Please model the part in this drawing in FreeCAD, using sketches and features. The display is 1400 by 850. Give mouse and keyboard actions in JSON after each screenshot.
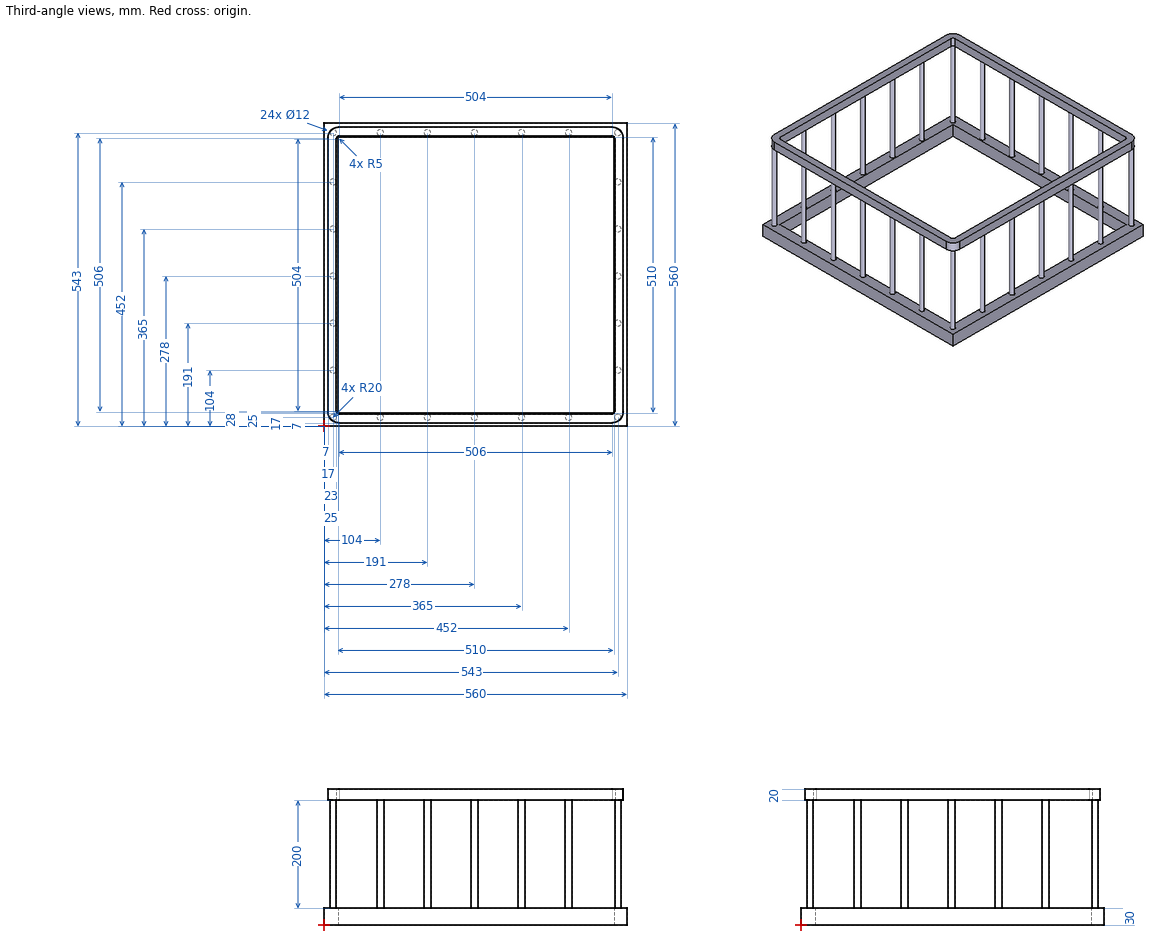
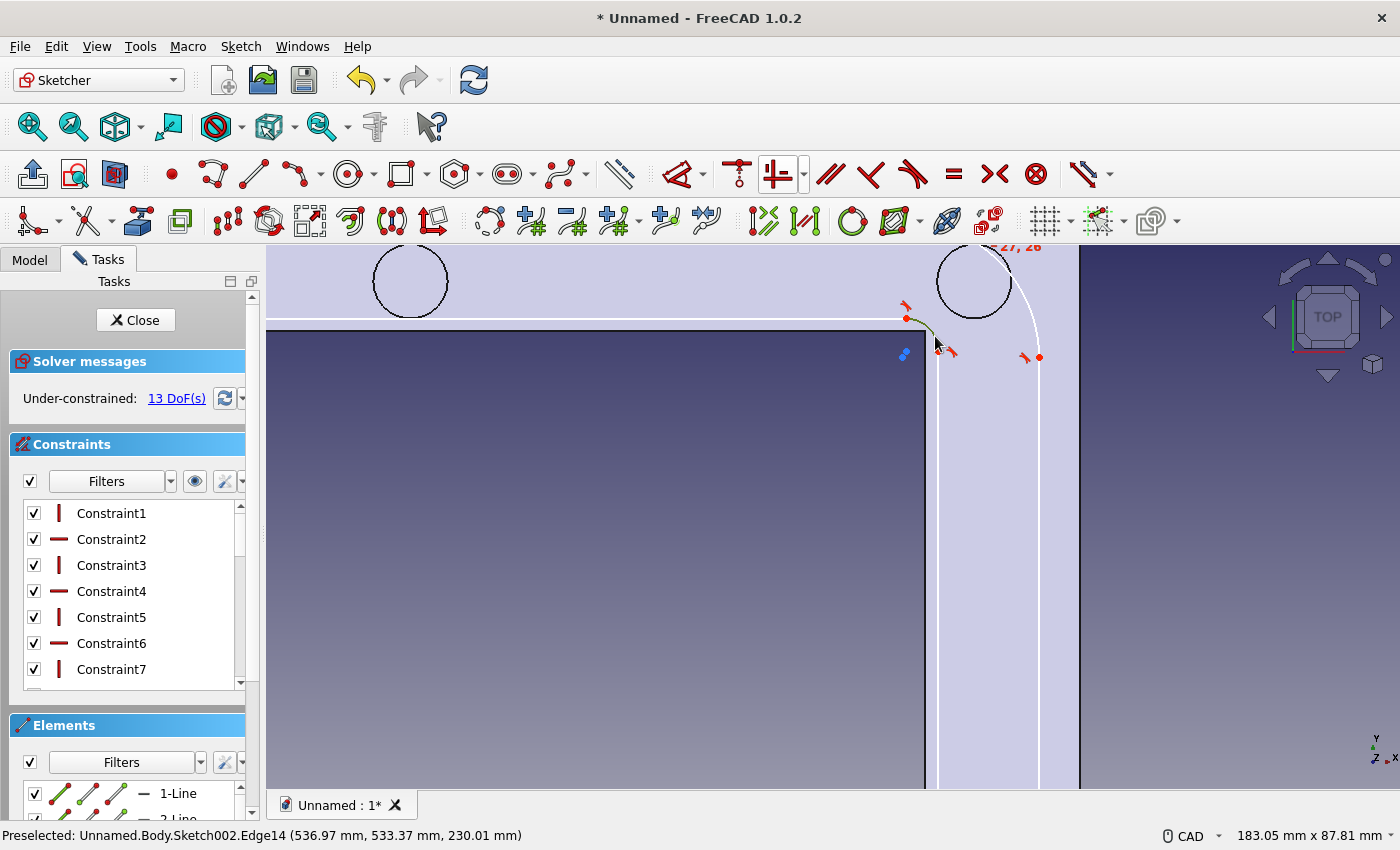
{"action": "scroll", "coordinate": [944, 341], "scroll_direction": "down", "scroll_amount": 11}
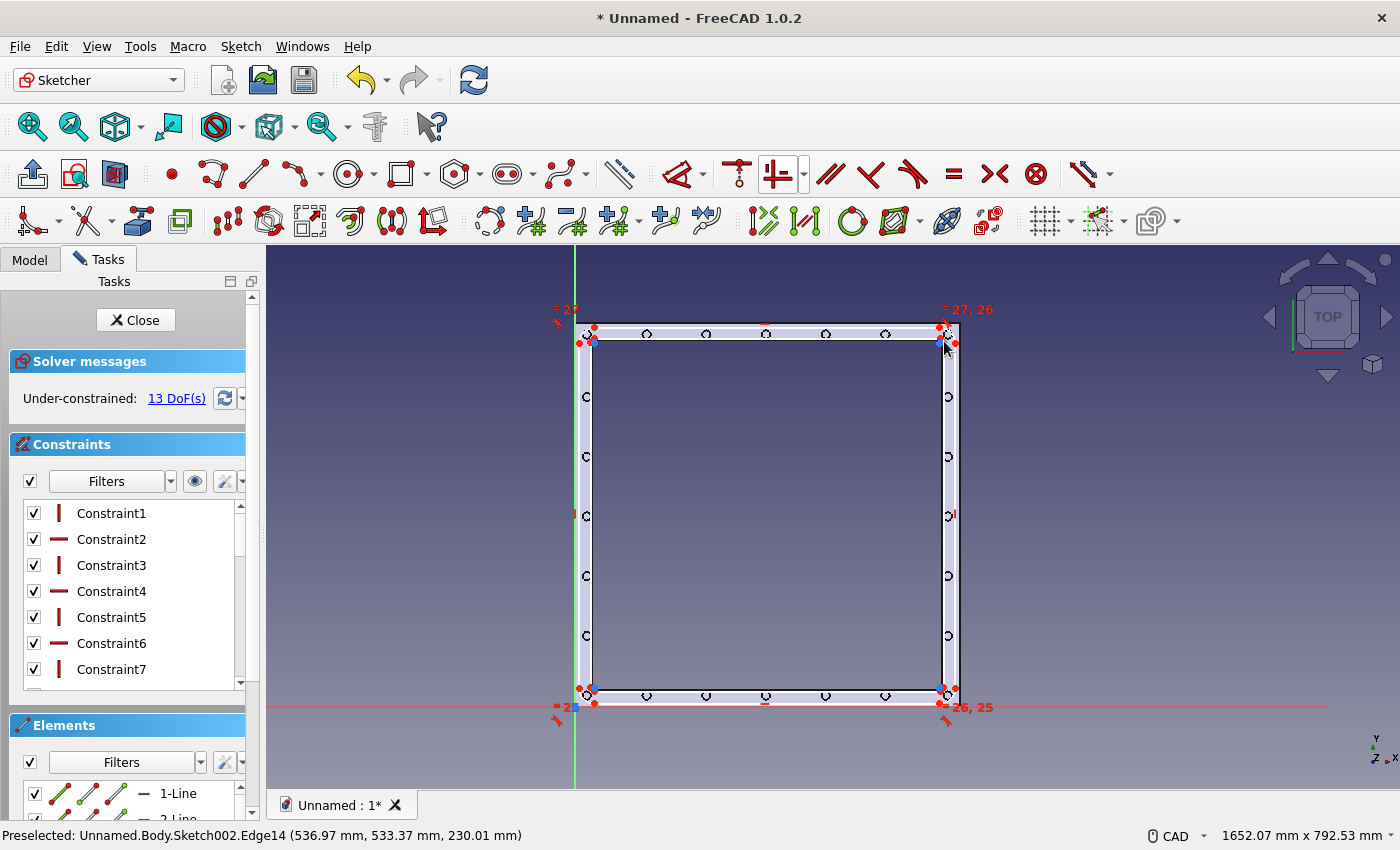
{"action": "scroll", "coordinate": [942, 691], "scroll_direction": "up", "scroll_amount": 11}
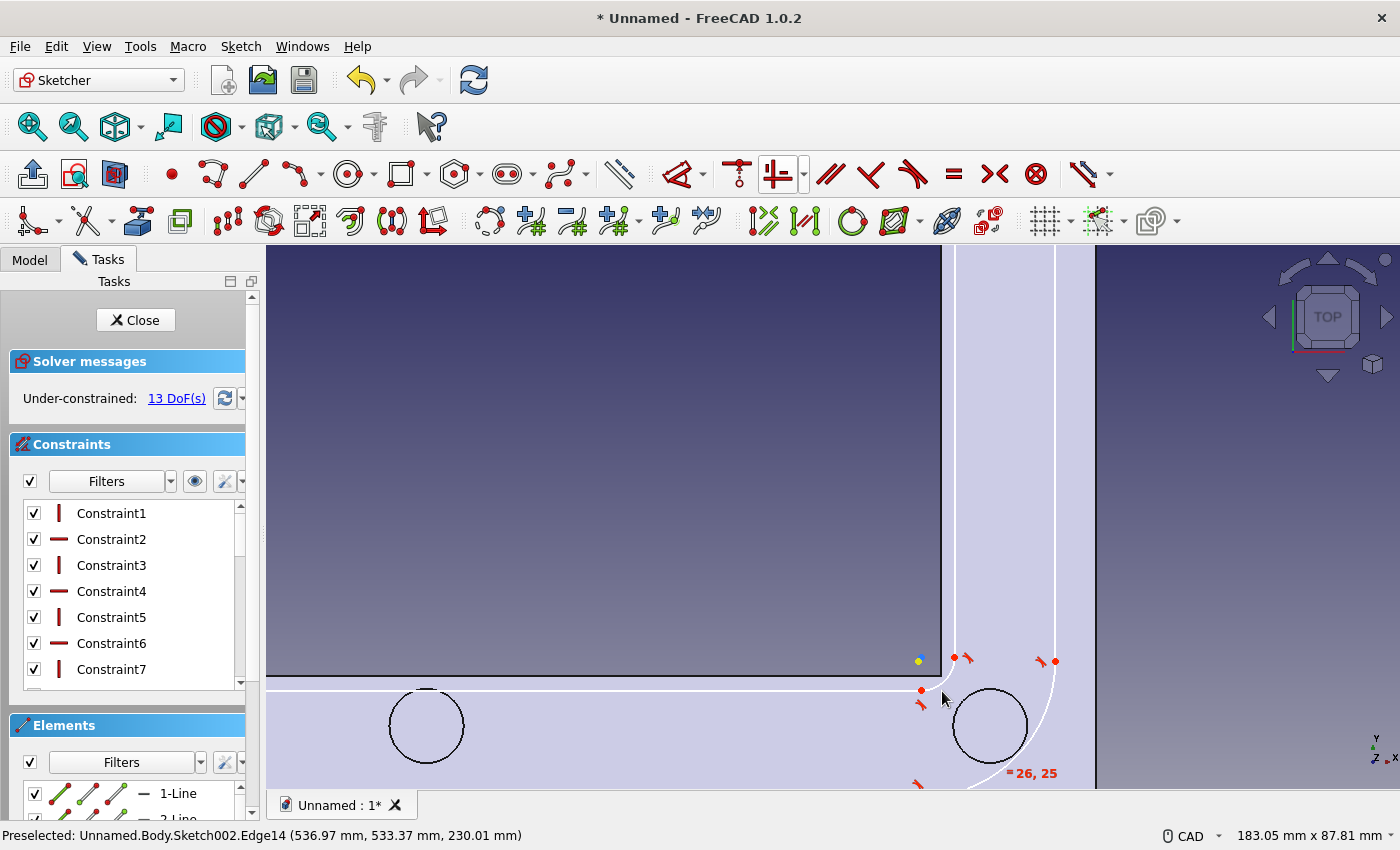
{"action": "left_click", "coordinate": [936, 687]}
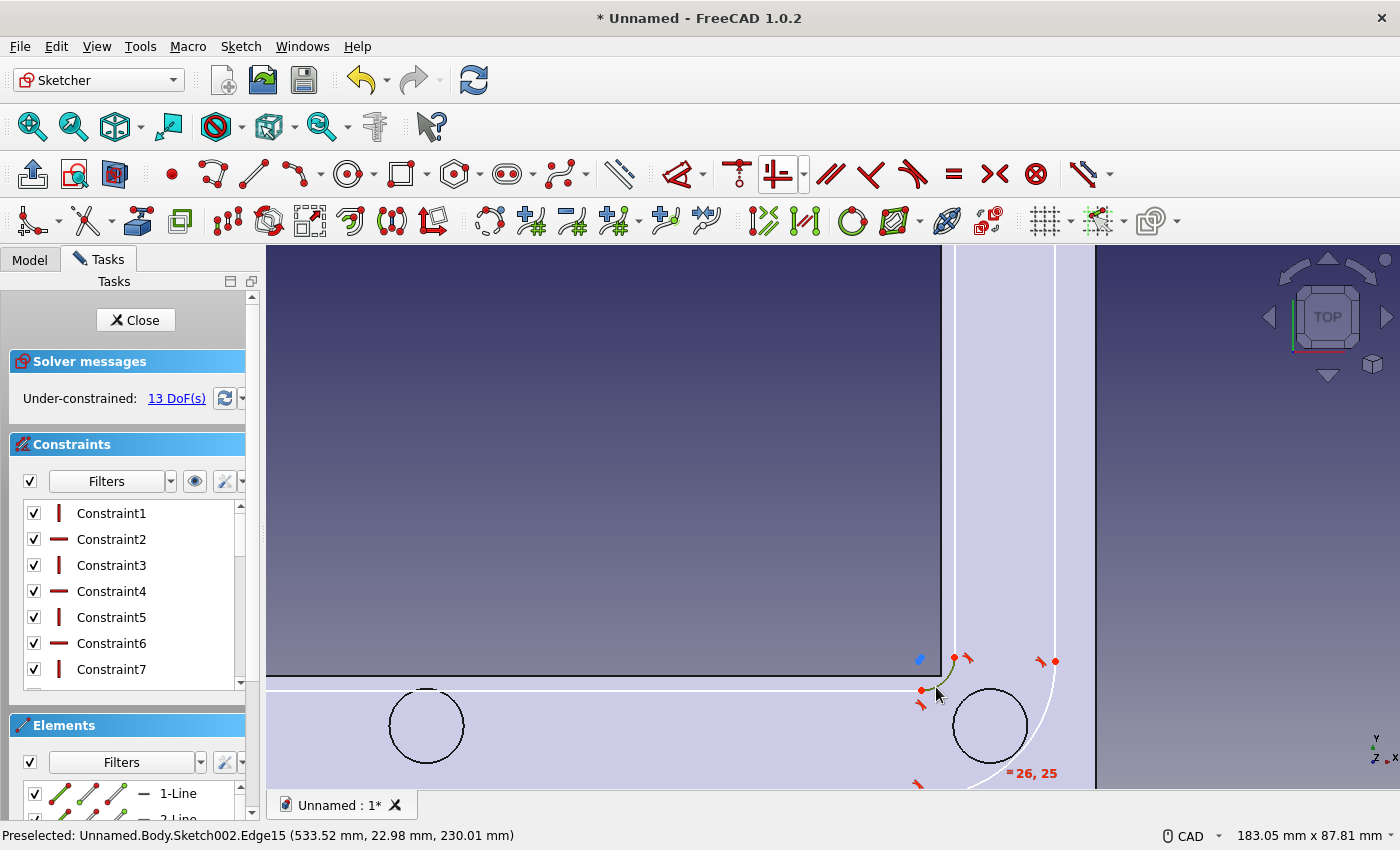
{"action": "scroll", "coordinate": [942, 691], "scroll_direction": "down", "scroll_amount": 11}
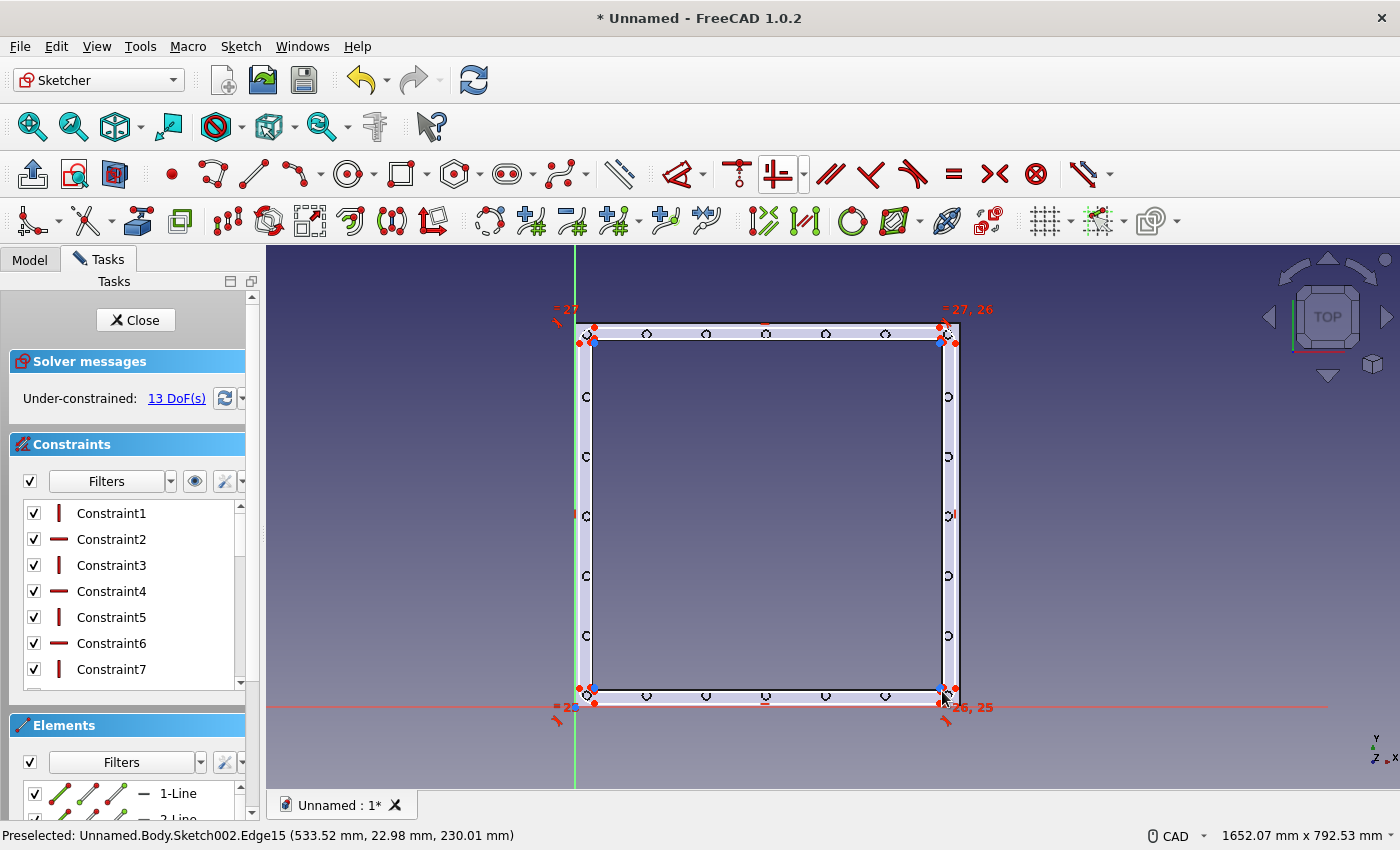
{"action": "scroll", "coordinate": [591, 690], "scroll_direction": "up", "scroll_amount": 11}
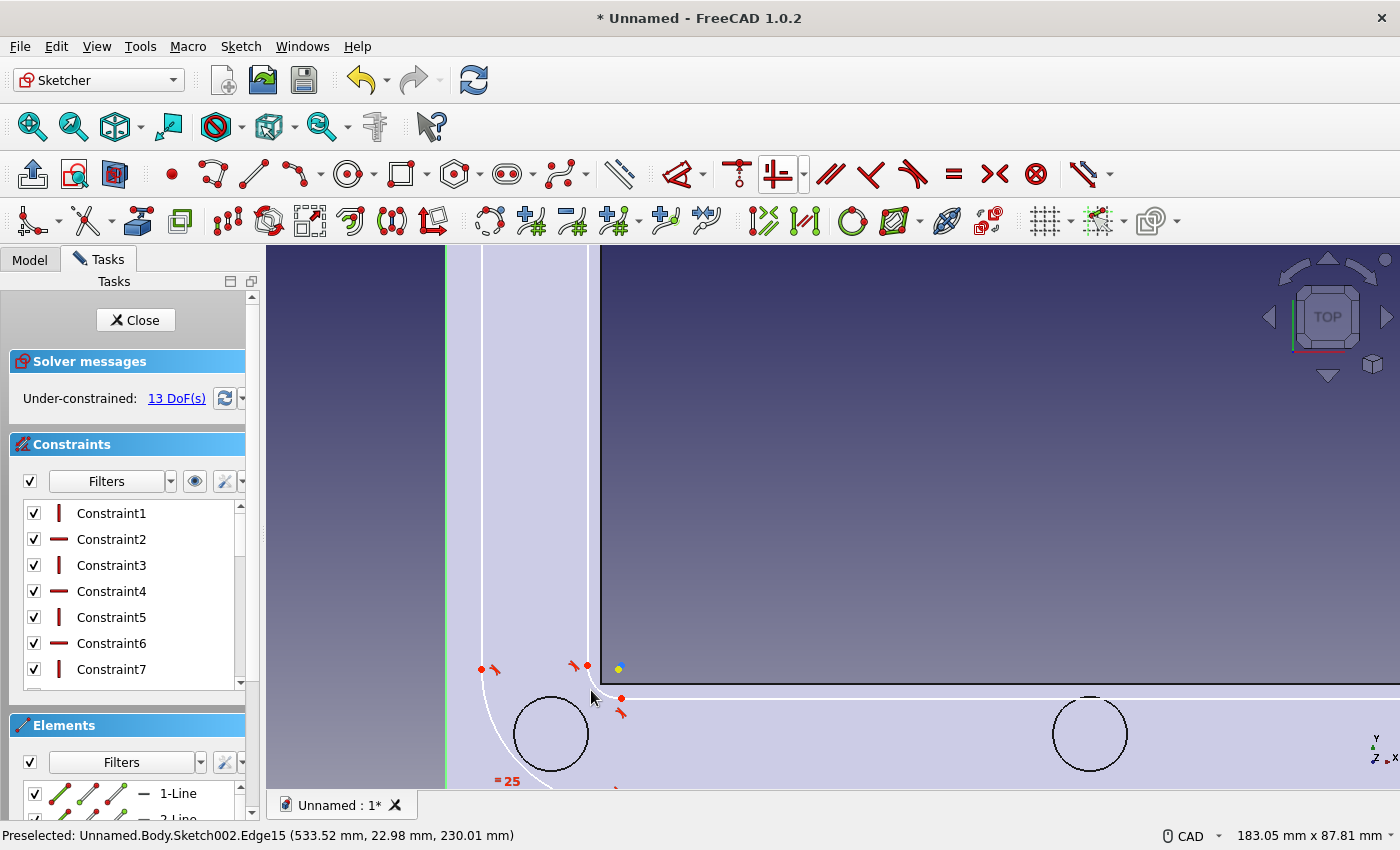
{"action": "left_click", "coordinate": [591, 680]}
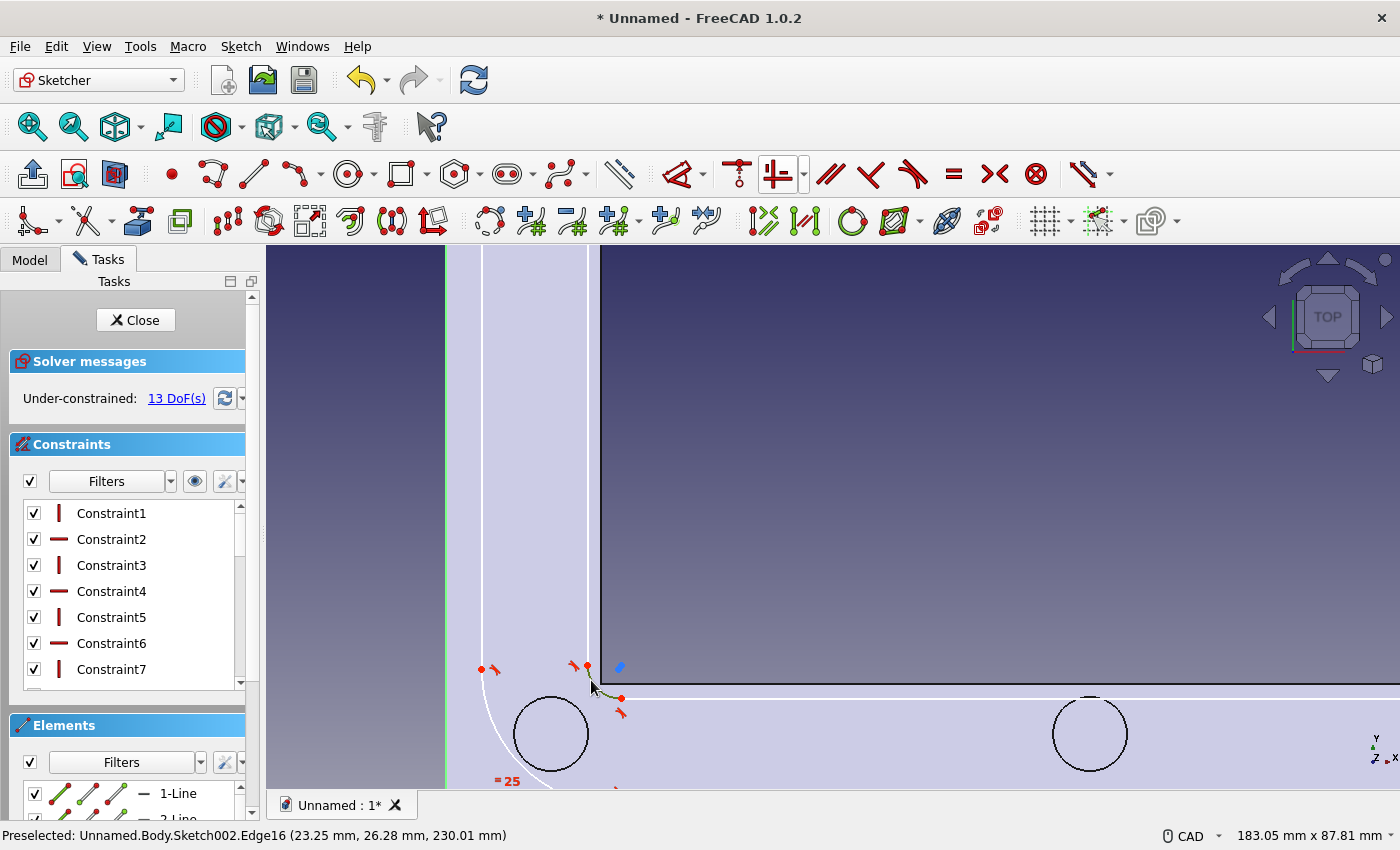
{"action": "left_click", "coordinate": [954, 174]}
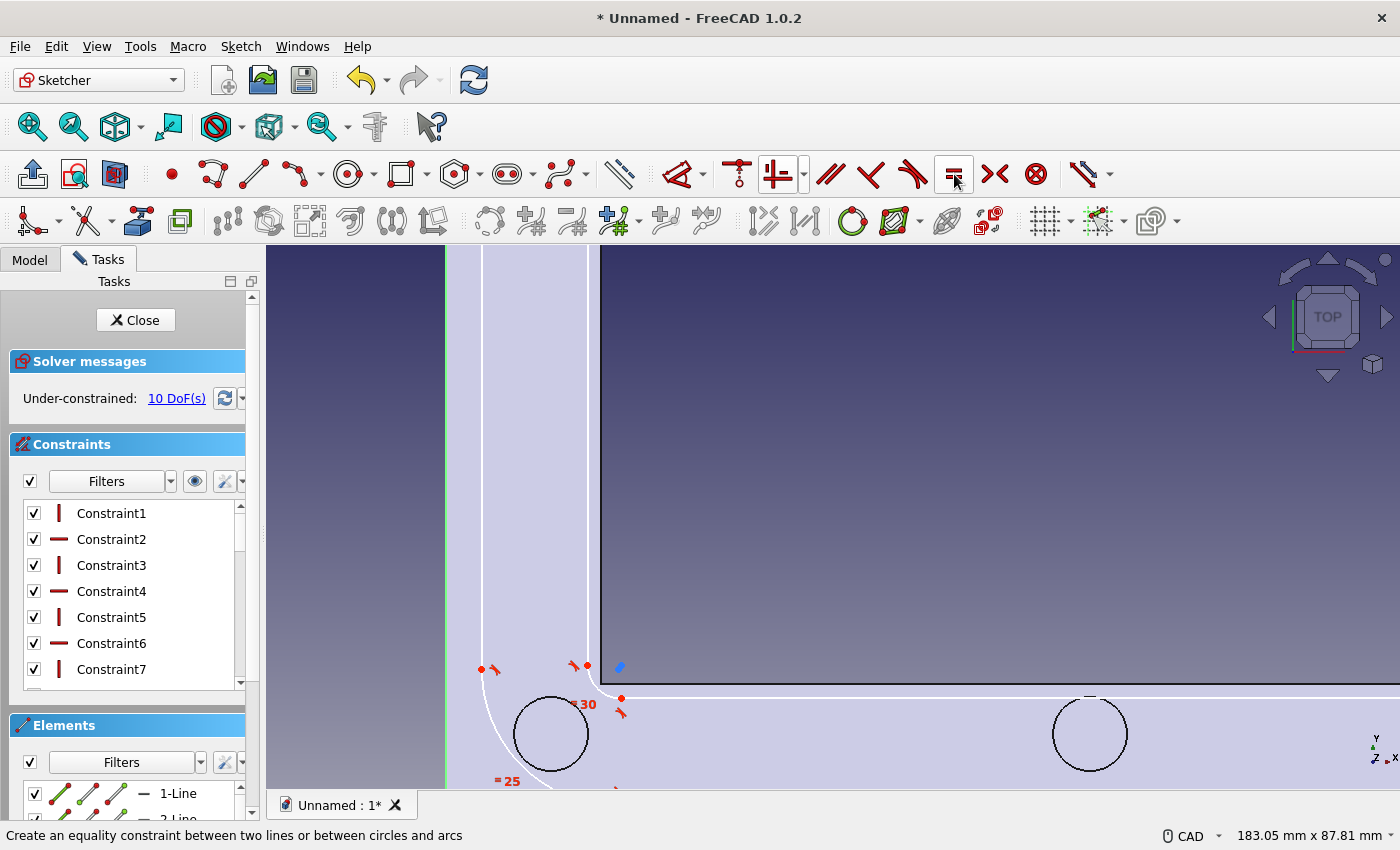
{"action": "left_click", "coordinate": [676, 174]}